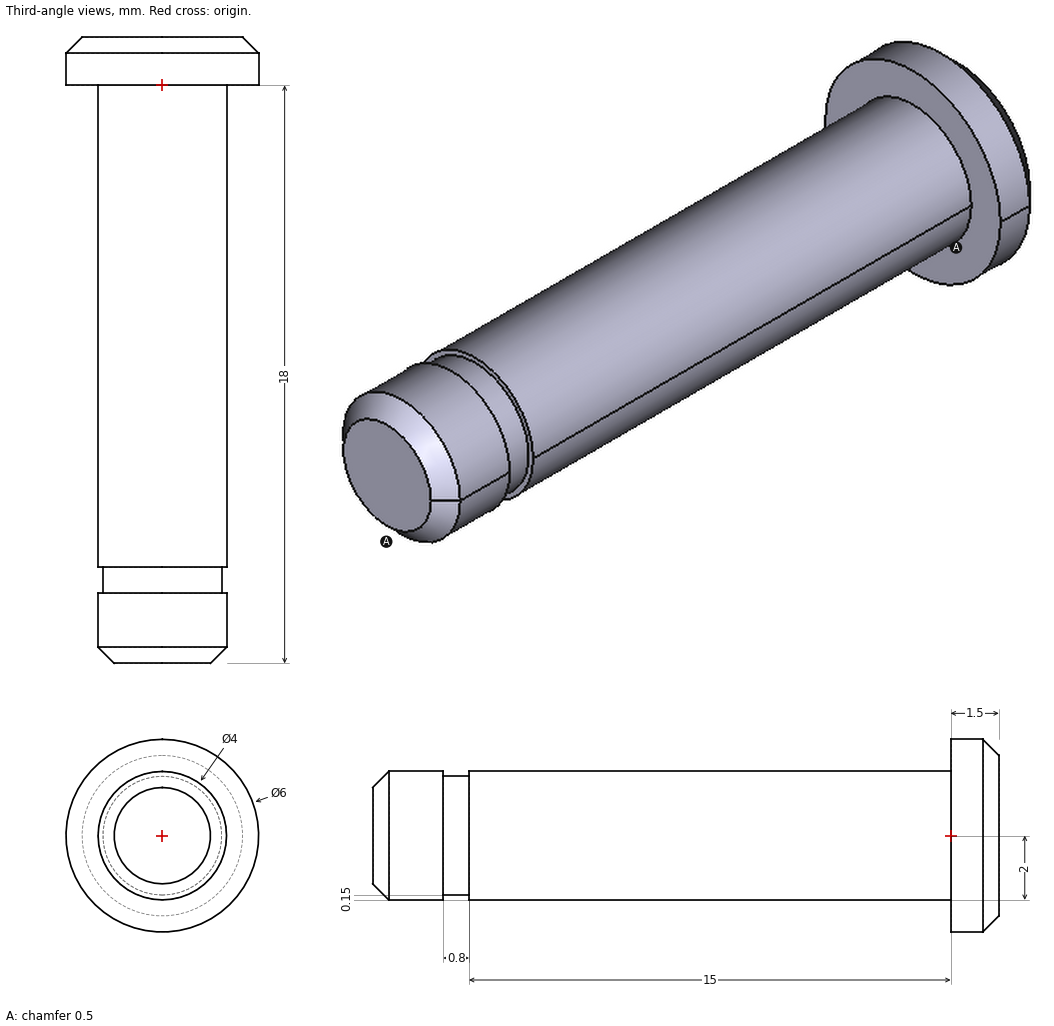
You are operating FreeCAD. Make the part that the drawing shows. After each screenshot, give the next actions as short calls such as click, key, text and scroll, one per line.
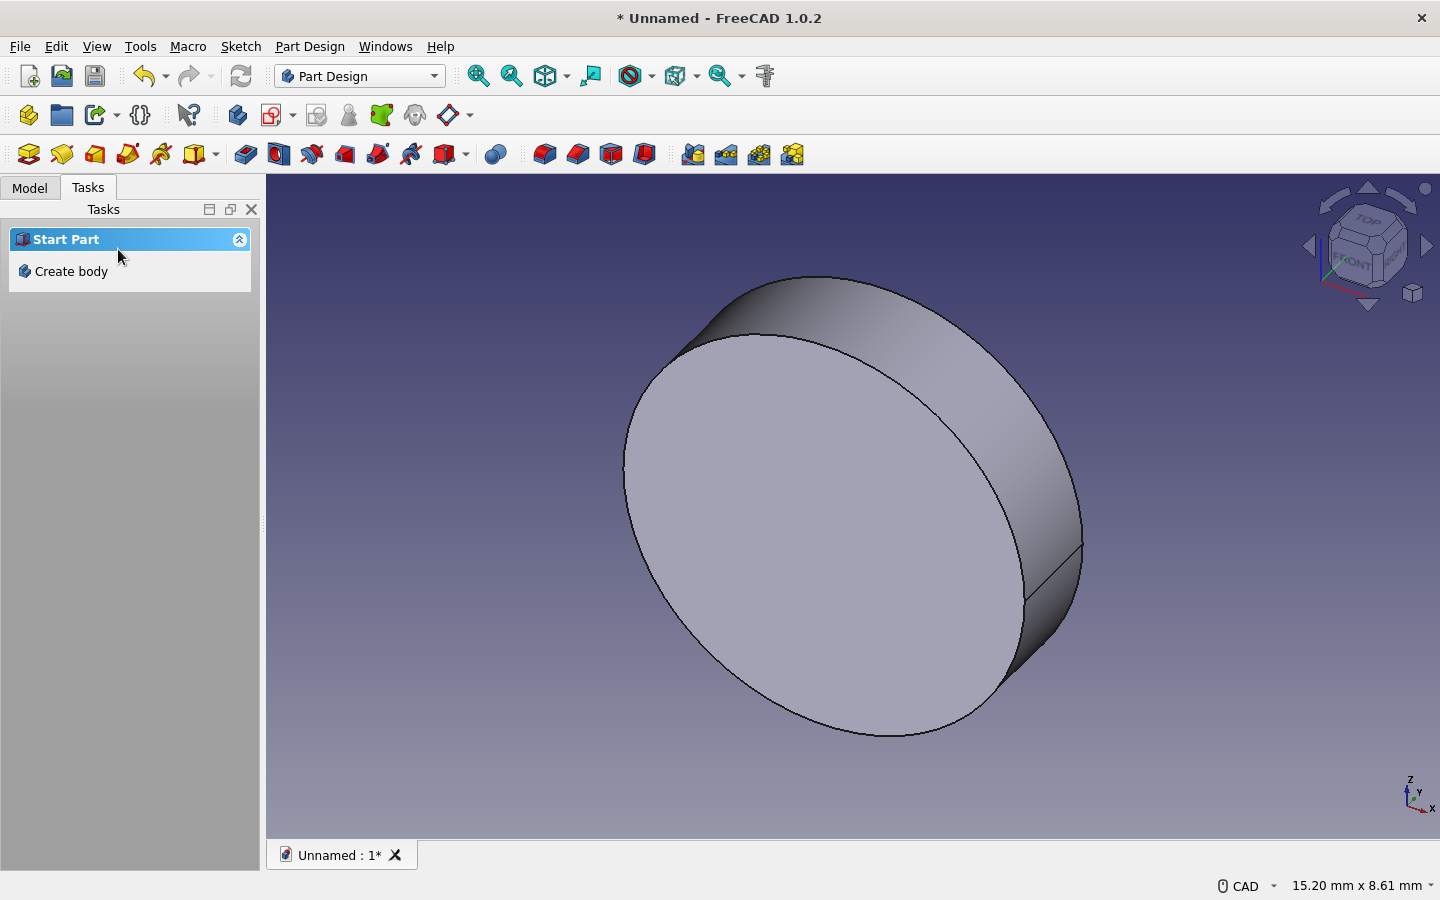
click(270, 116)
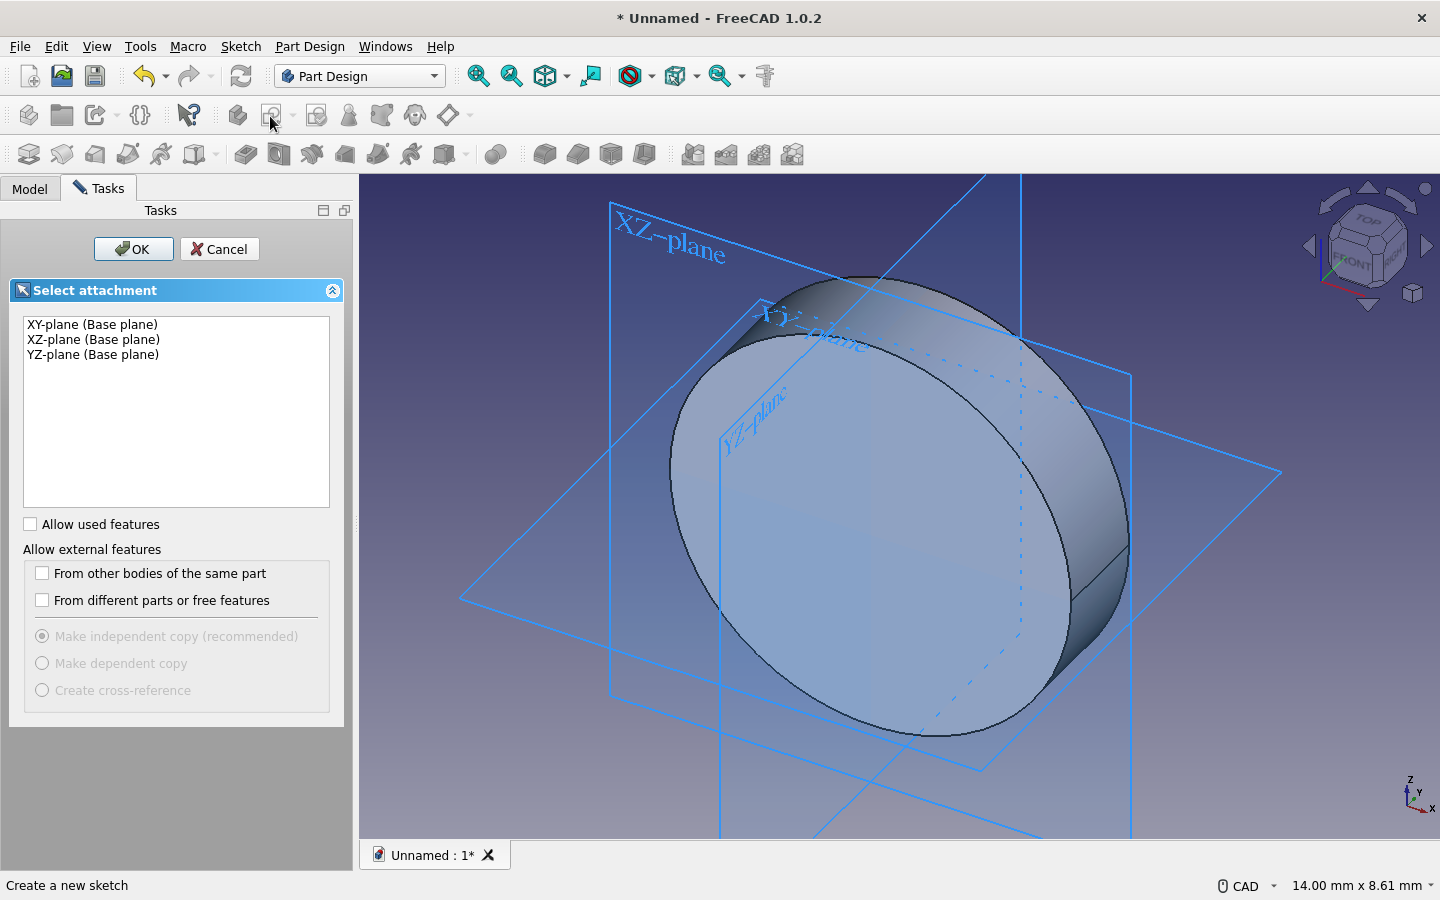
click(84, 340)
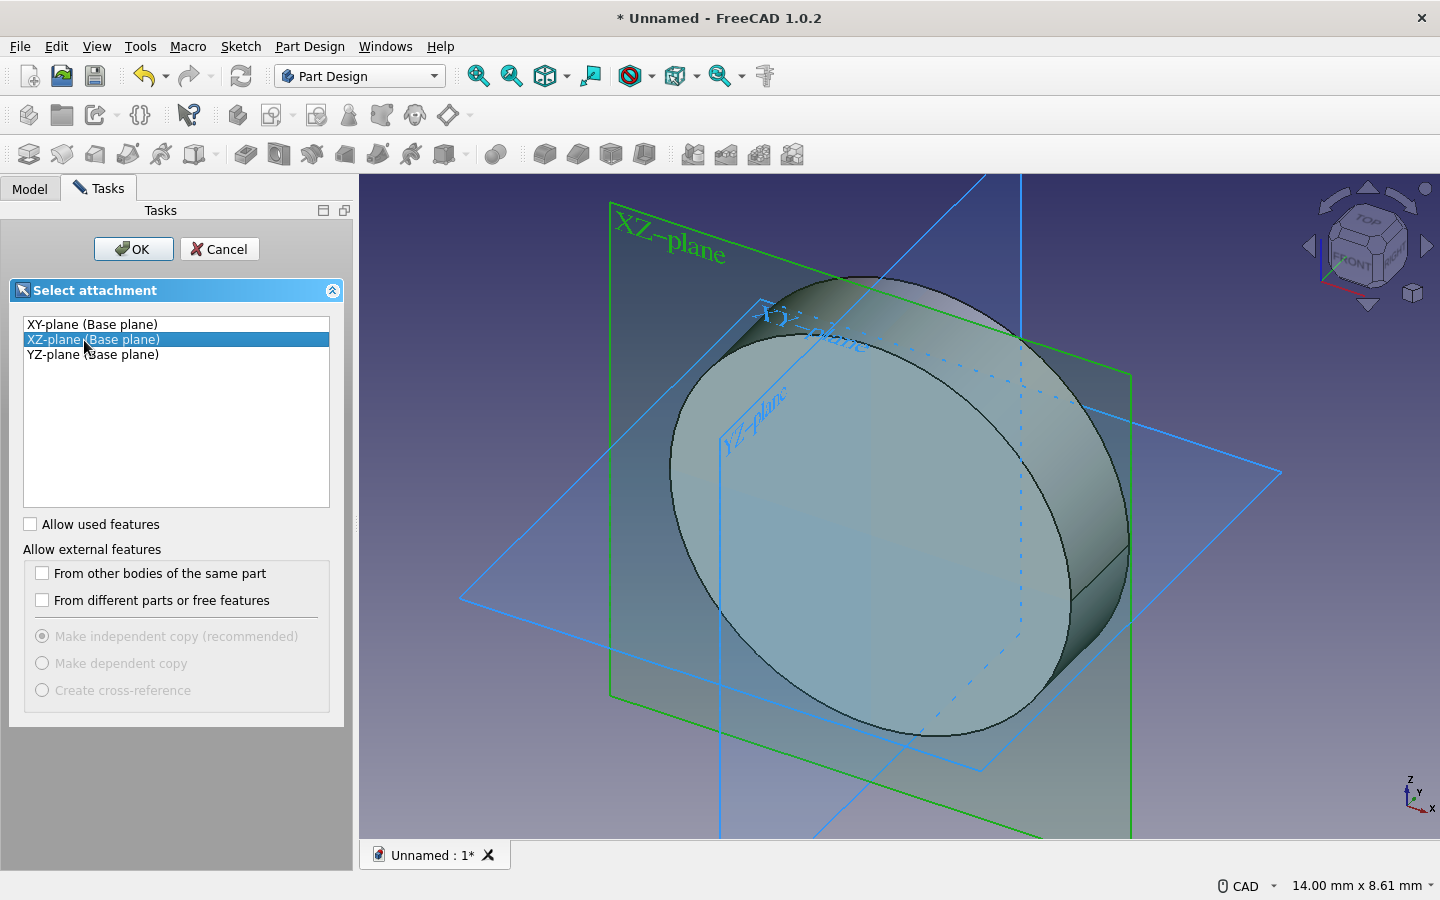
click(134, 249)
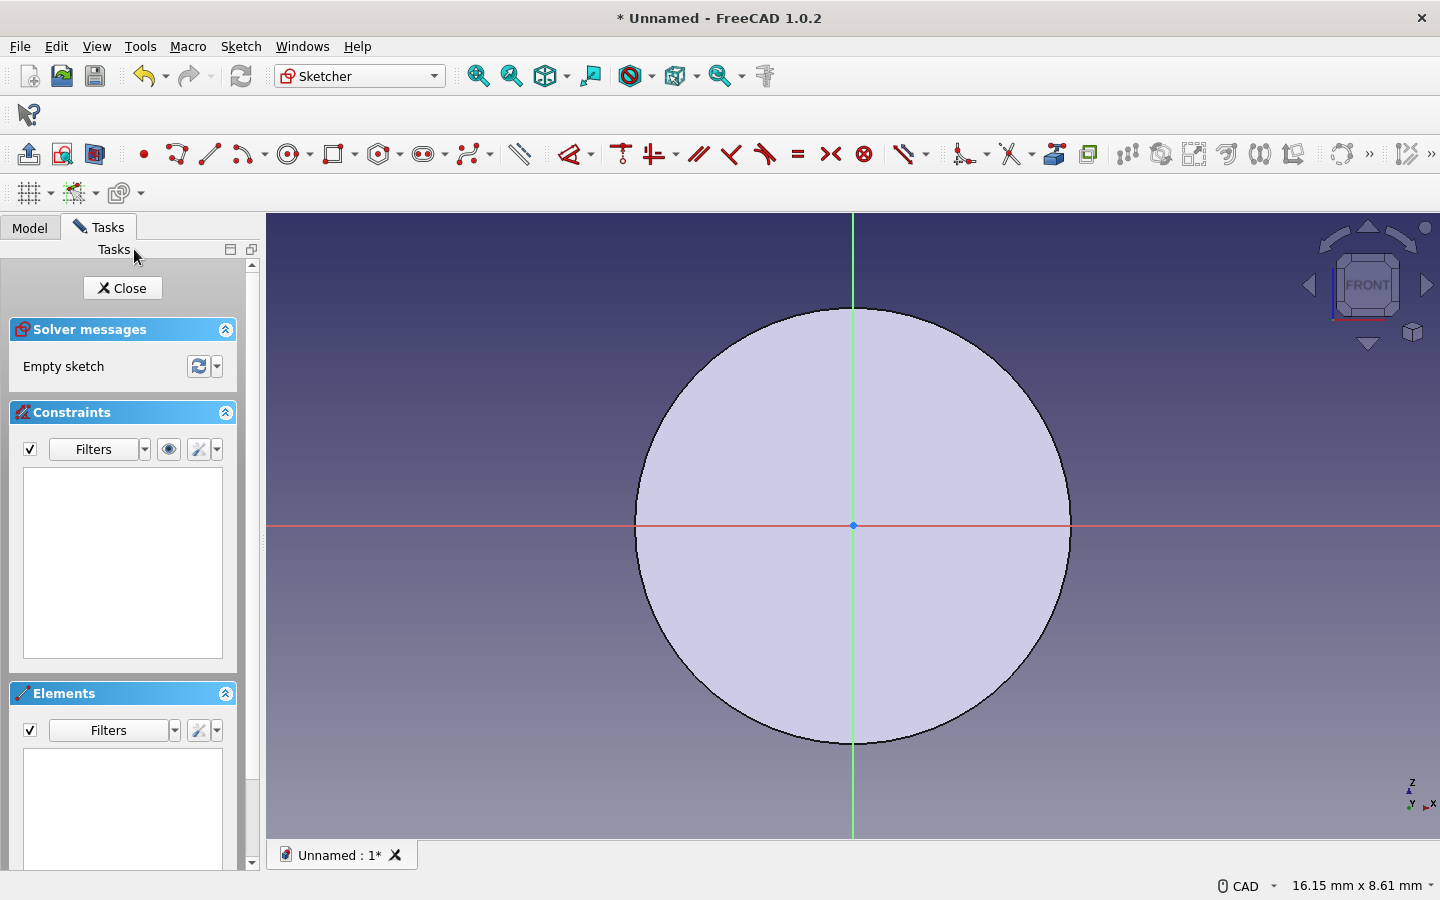
scroll(992, 526, up, 2)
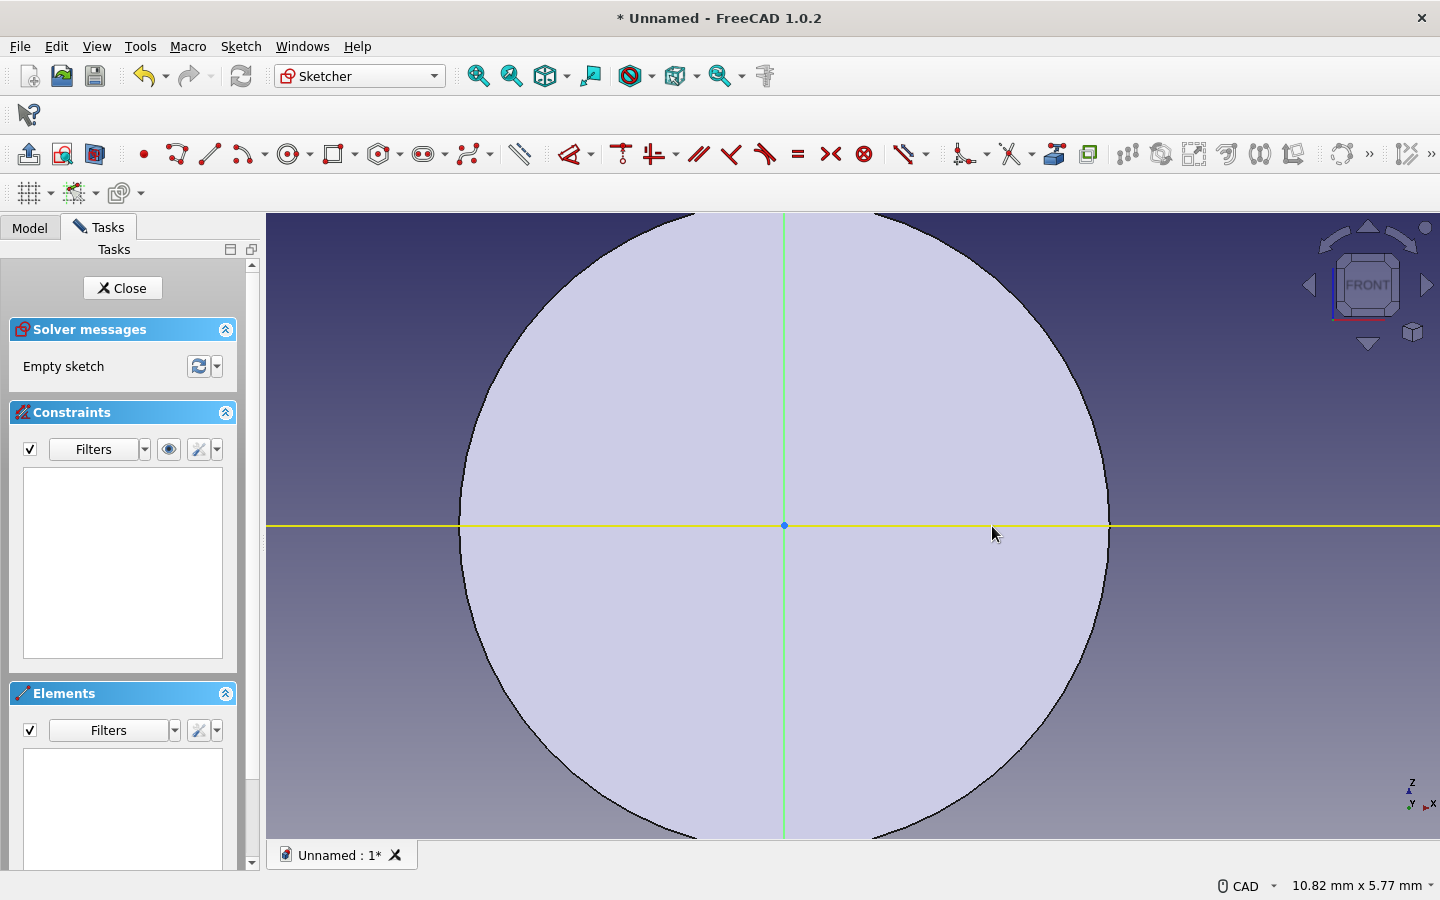
click(288, 154)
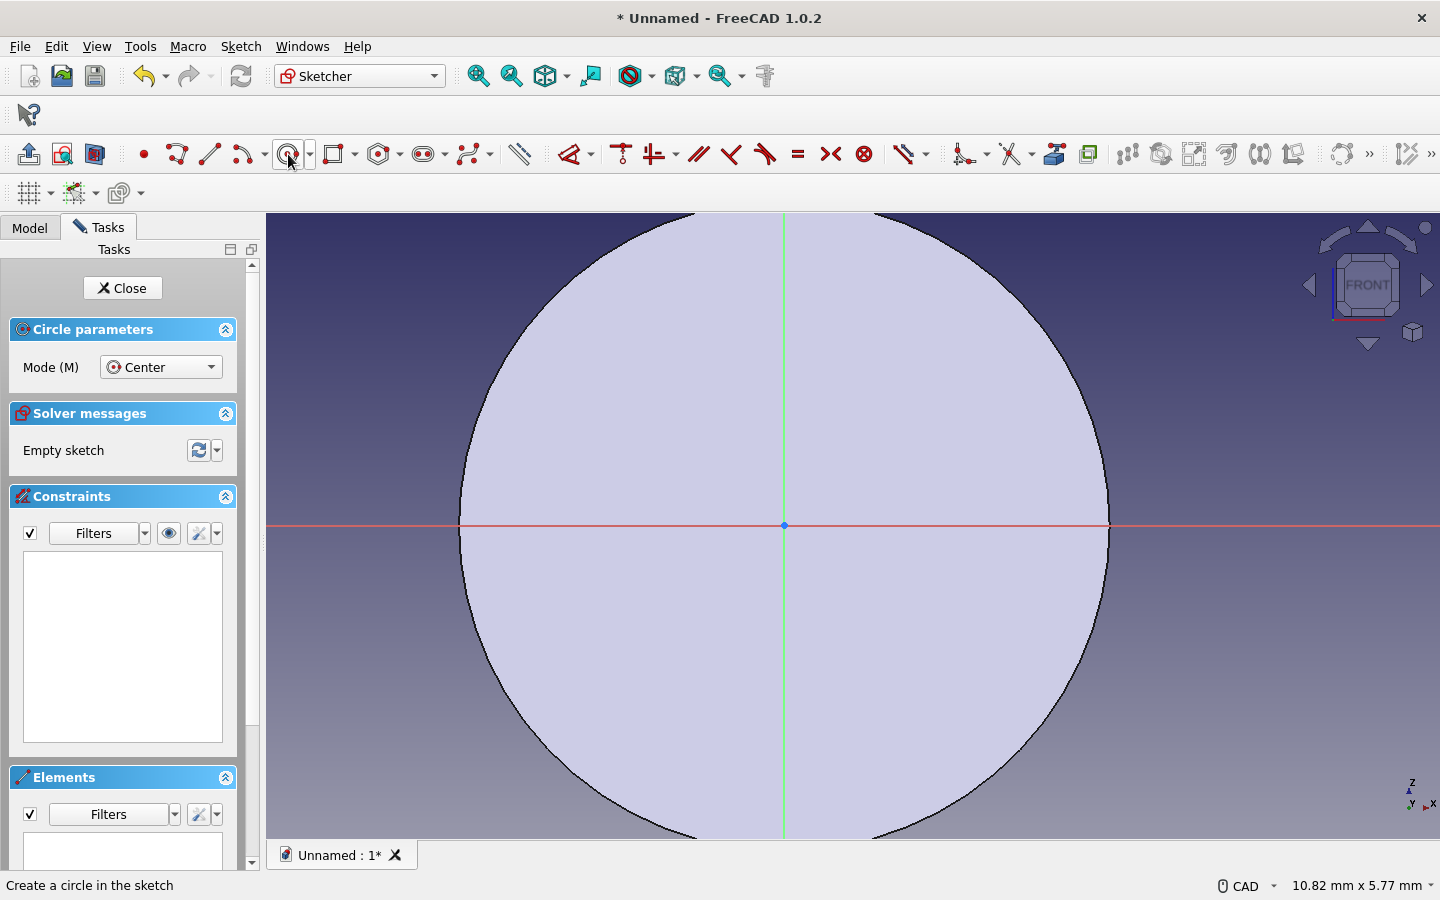
click(784, 526)
move(938, 372)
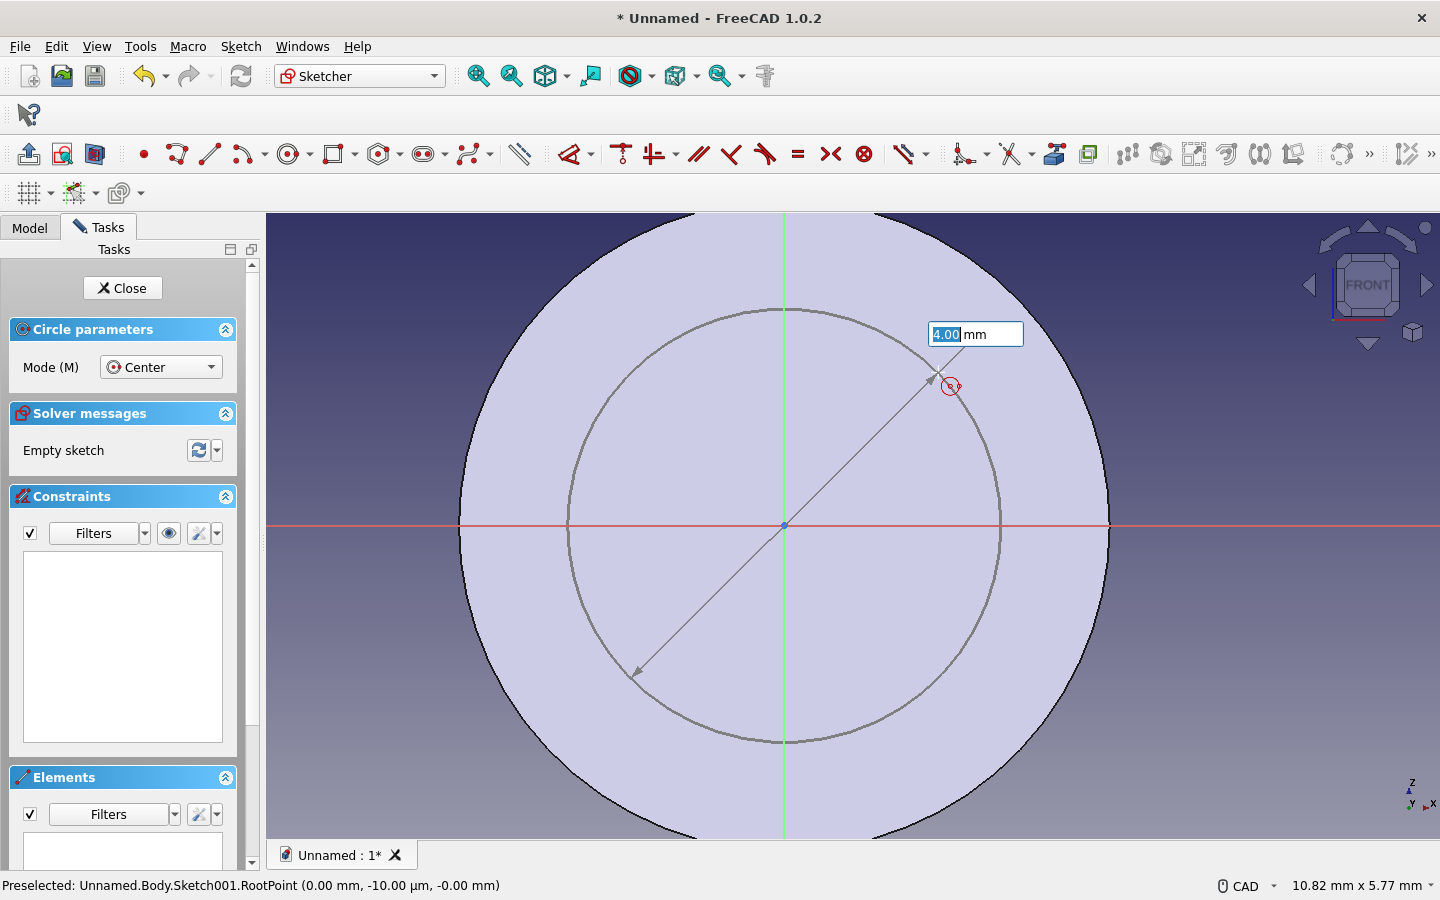
text(4)
key(Return)
key(Escape)